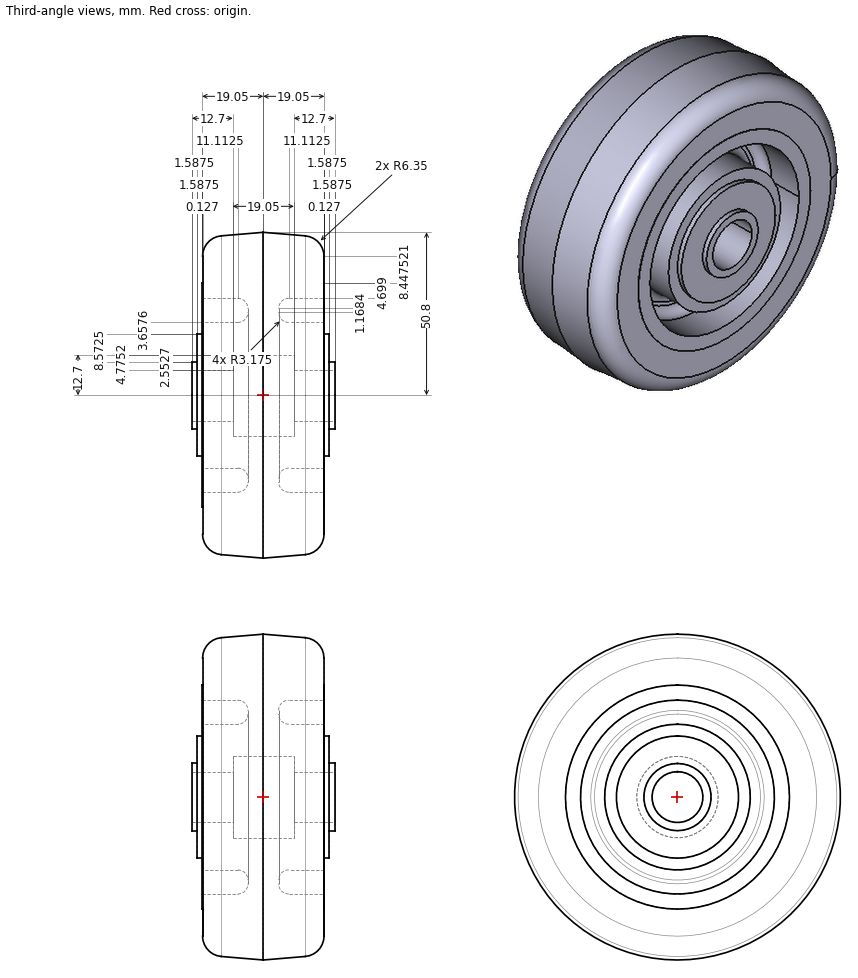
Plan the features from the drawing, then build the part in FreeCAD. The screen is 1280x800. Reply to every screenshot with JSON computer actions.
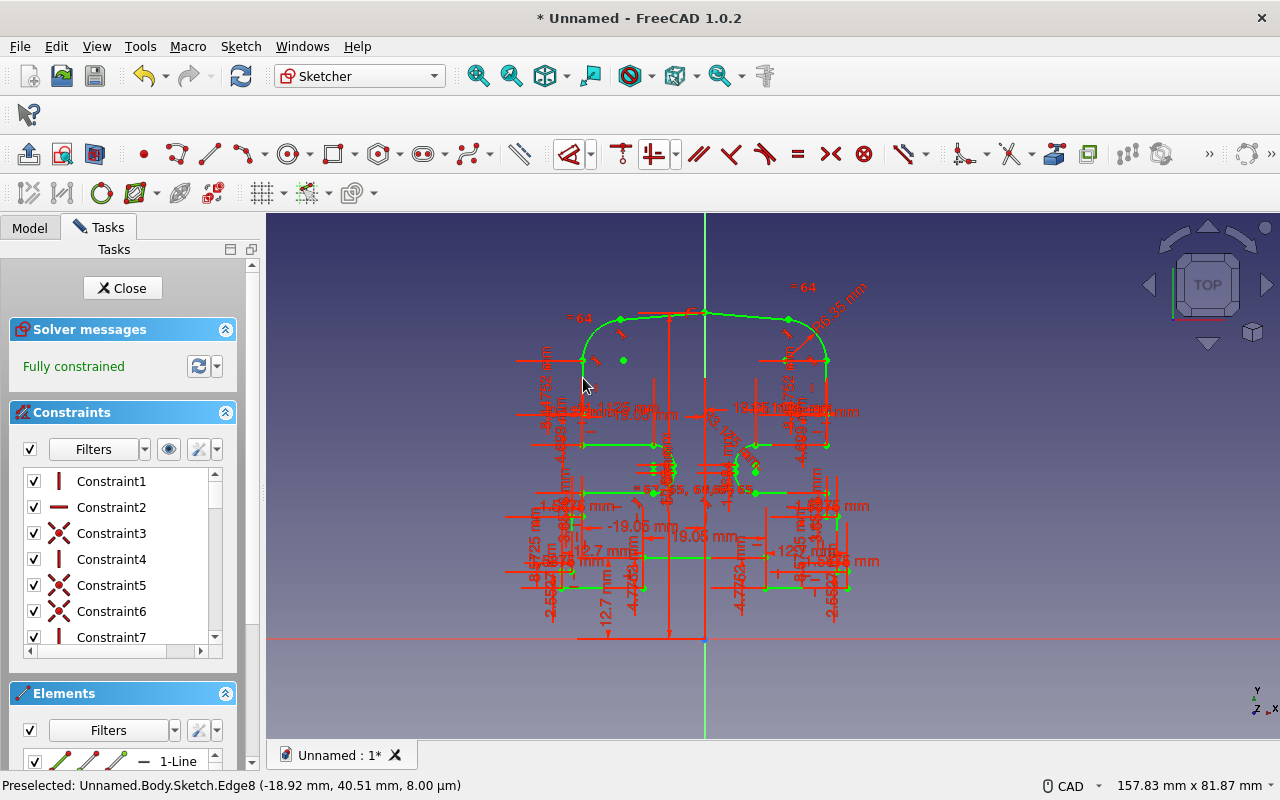
{"action": "left_click", "coordinate": [123, 288]}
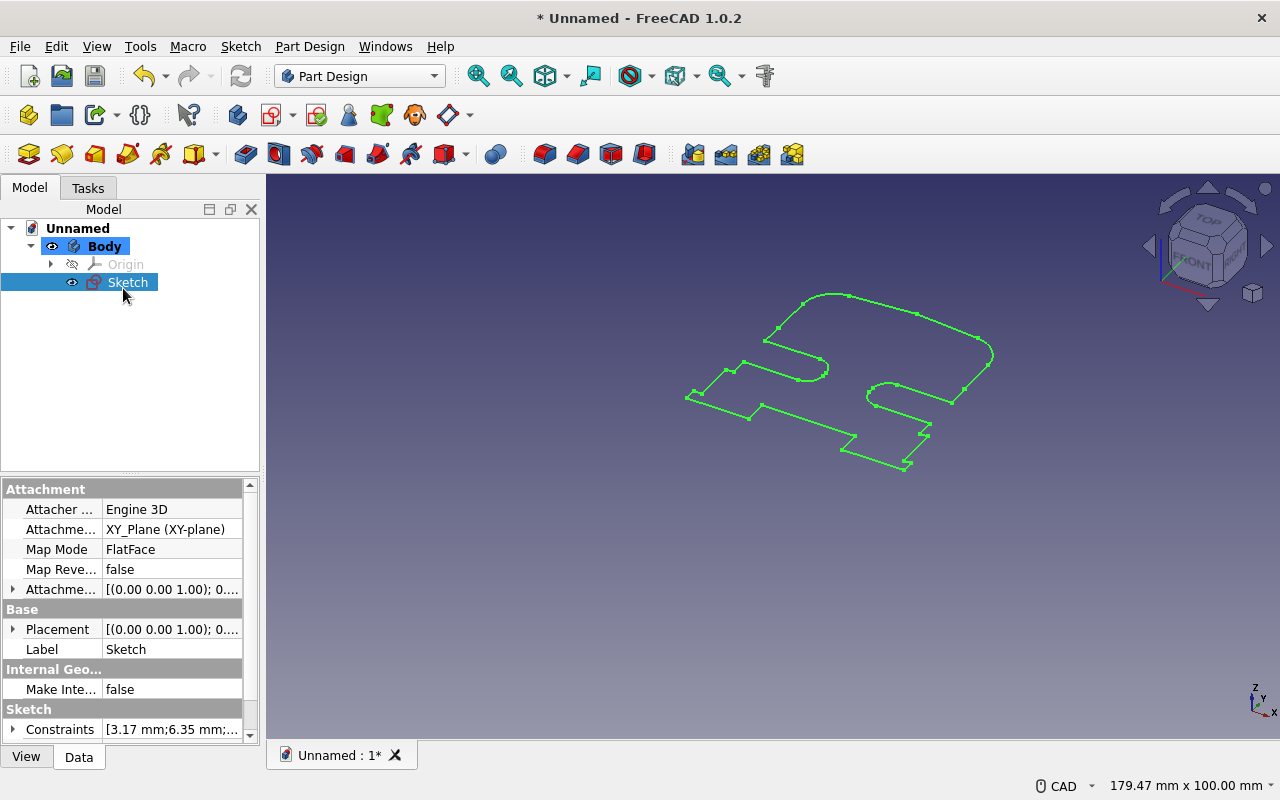
{"action": "left_click", "coordinate": [62, 154]}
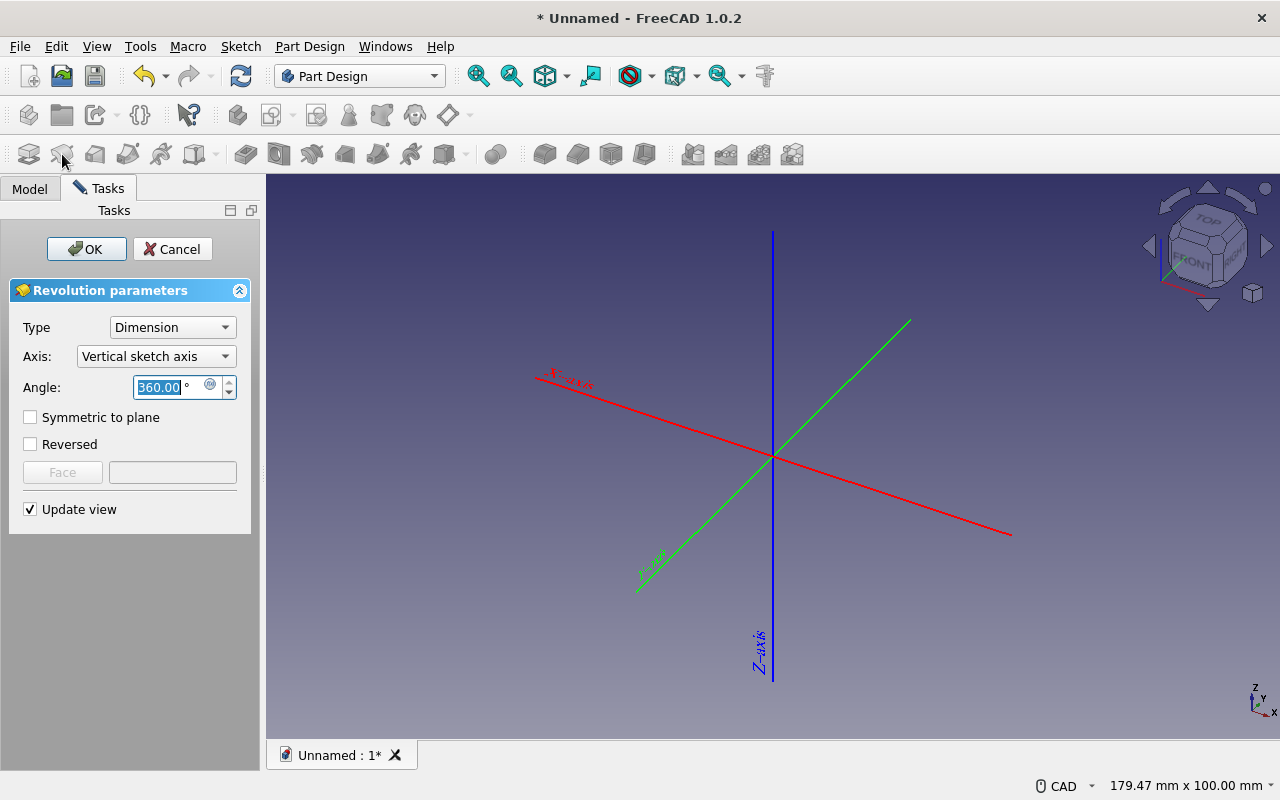
{"action": "left_click", "coordinate": [157, 356]}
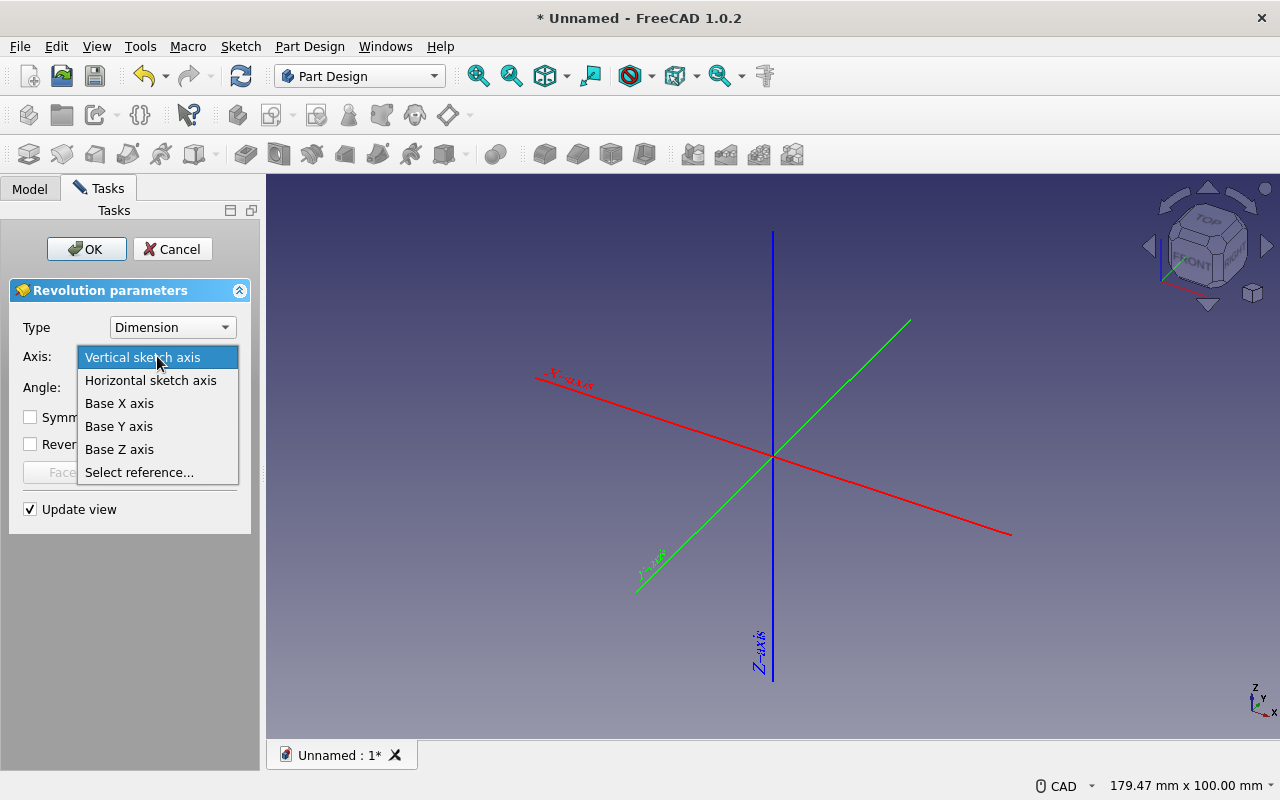
{"action": "left_click", "coordinate": [156, 380]}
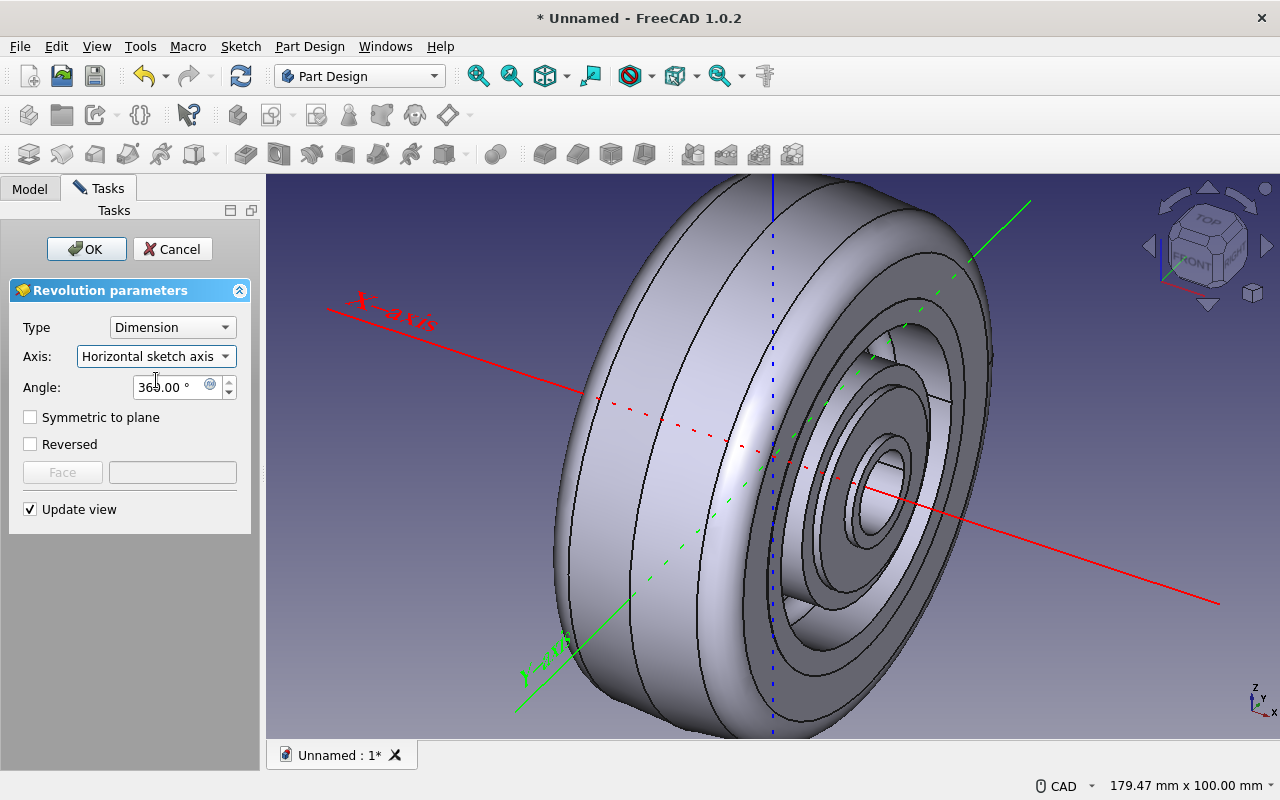
{"action": "left_click", "coordinate": [87, 249]}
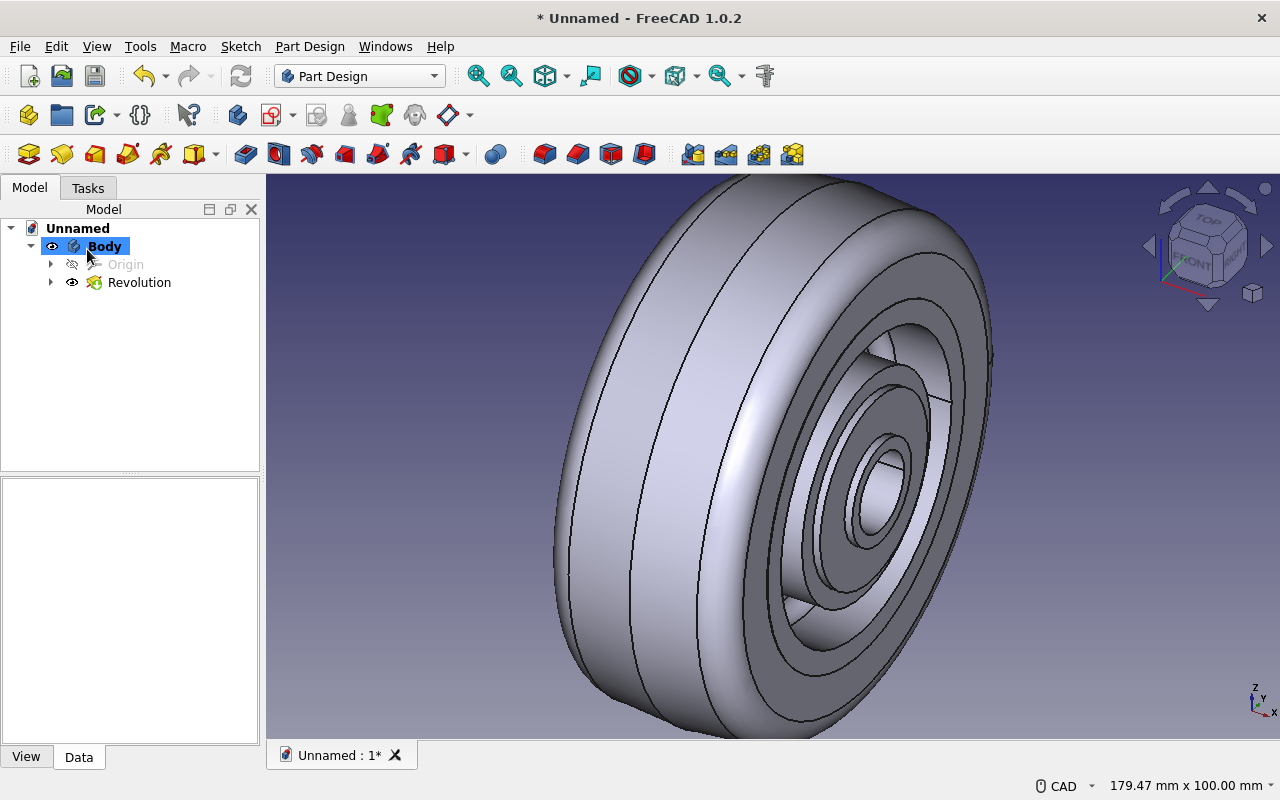
{"action": "key", "text": "0"}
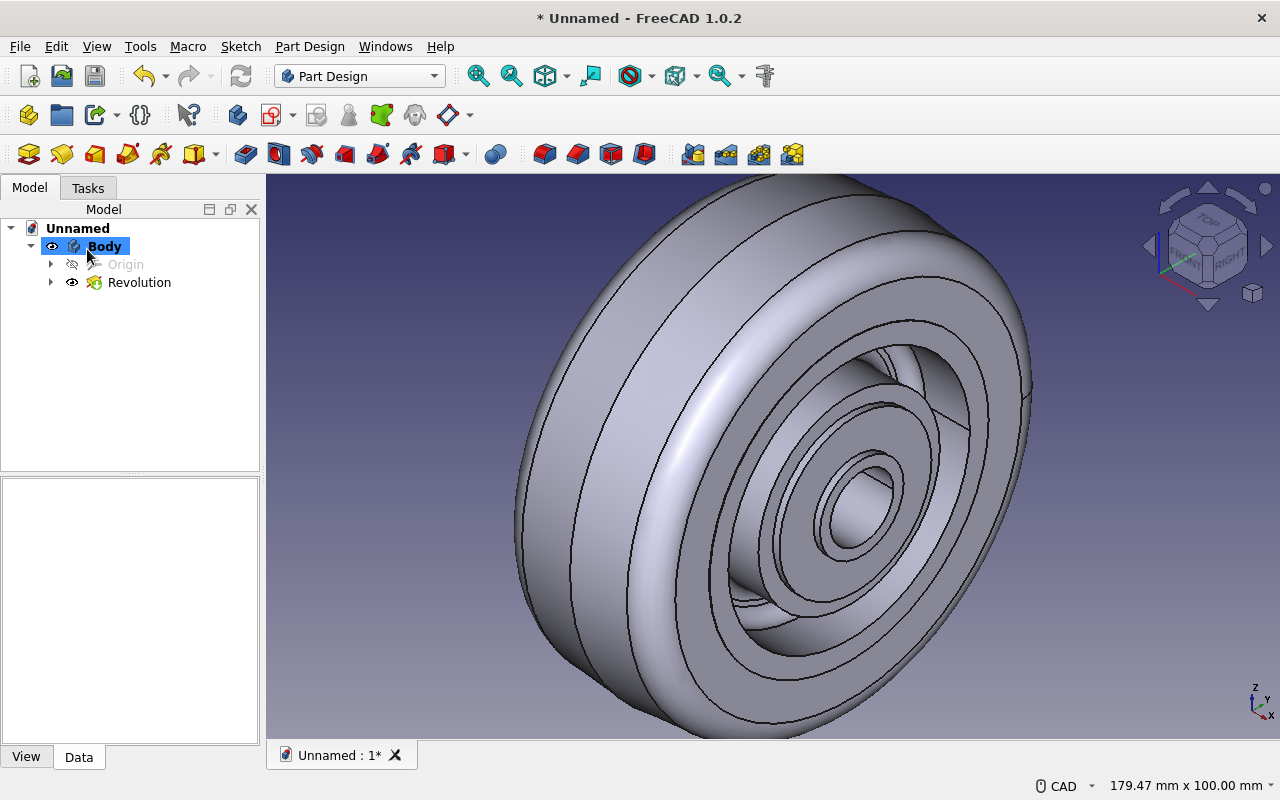
{"action": "left_click", "coordinate": [479, 76]}